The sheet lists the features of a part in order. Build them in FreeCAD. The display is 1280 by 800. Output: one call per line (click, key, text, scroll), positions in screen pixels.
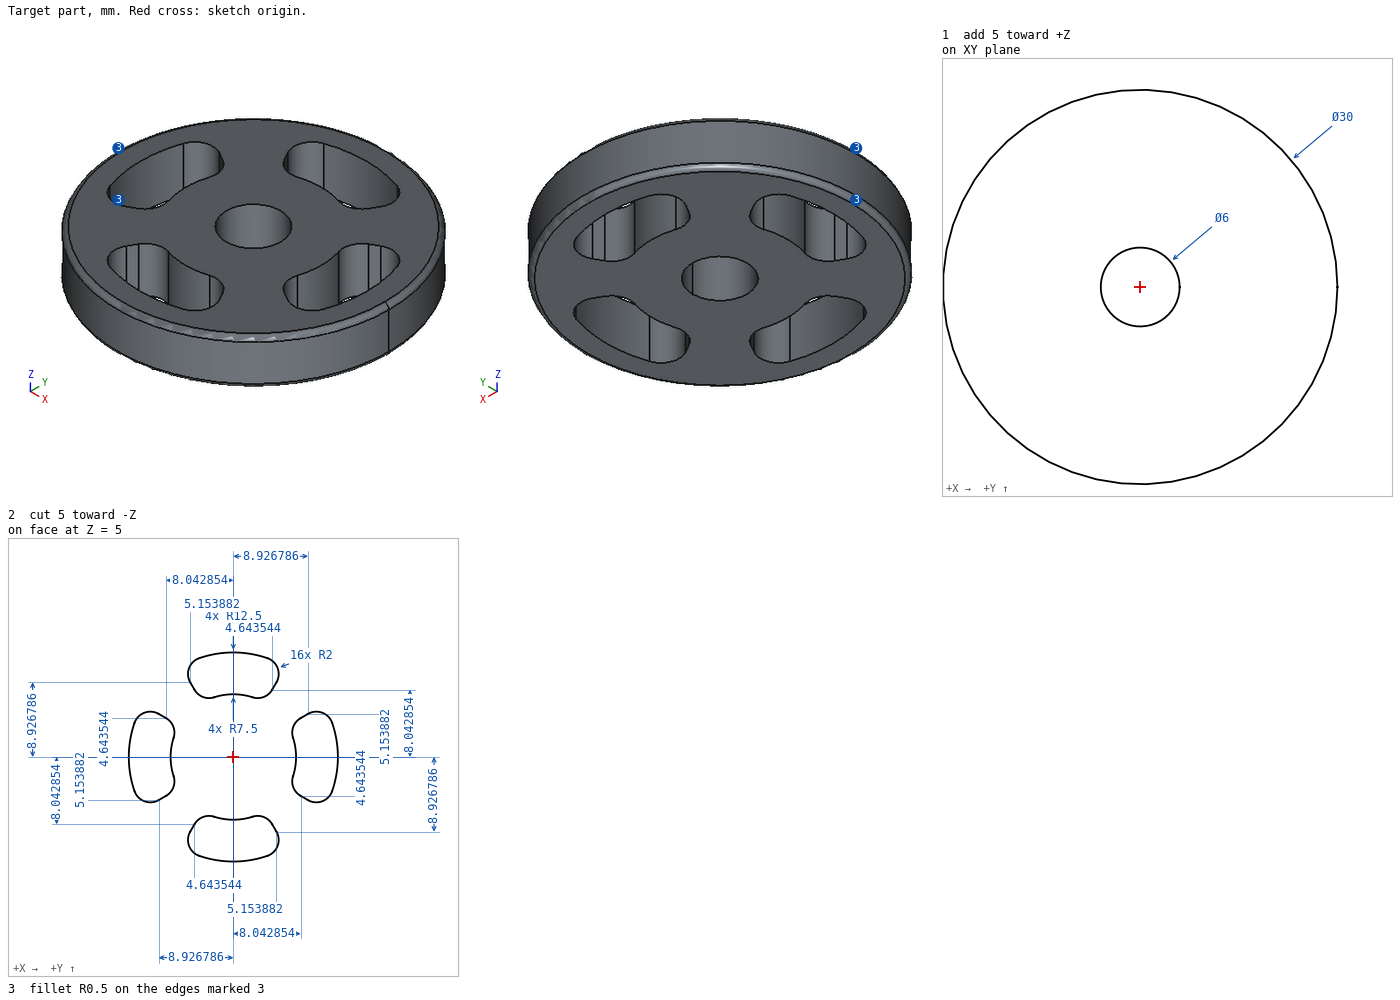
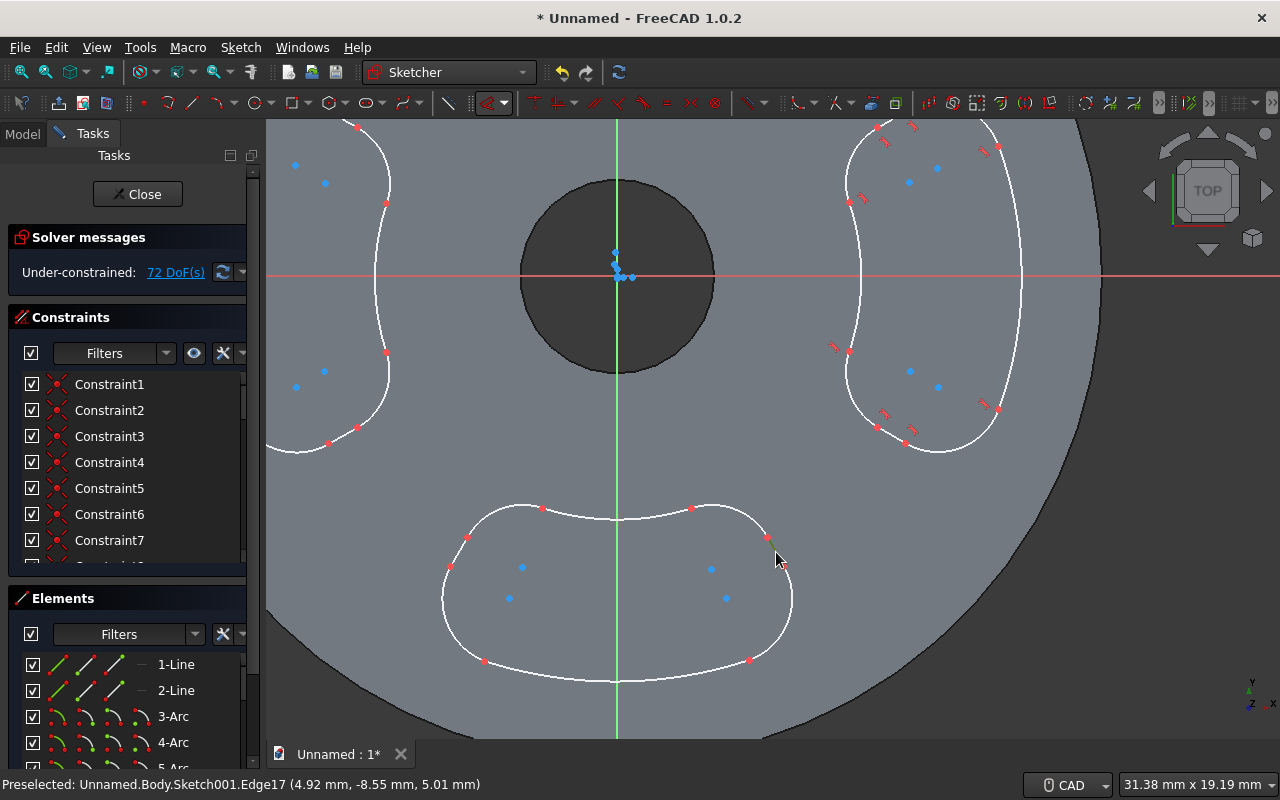
click(750, 518)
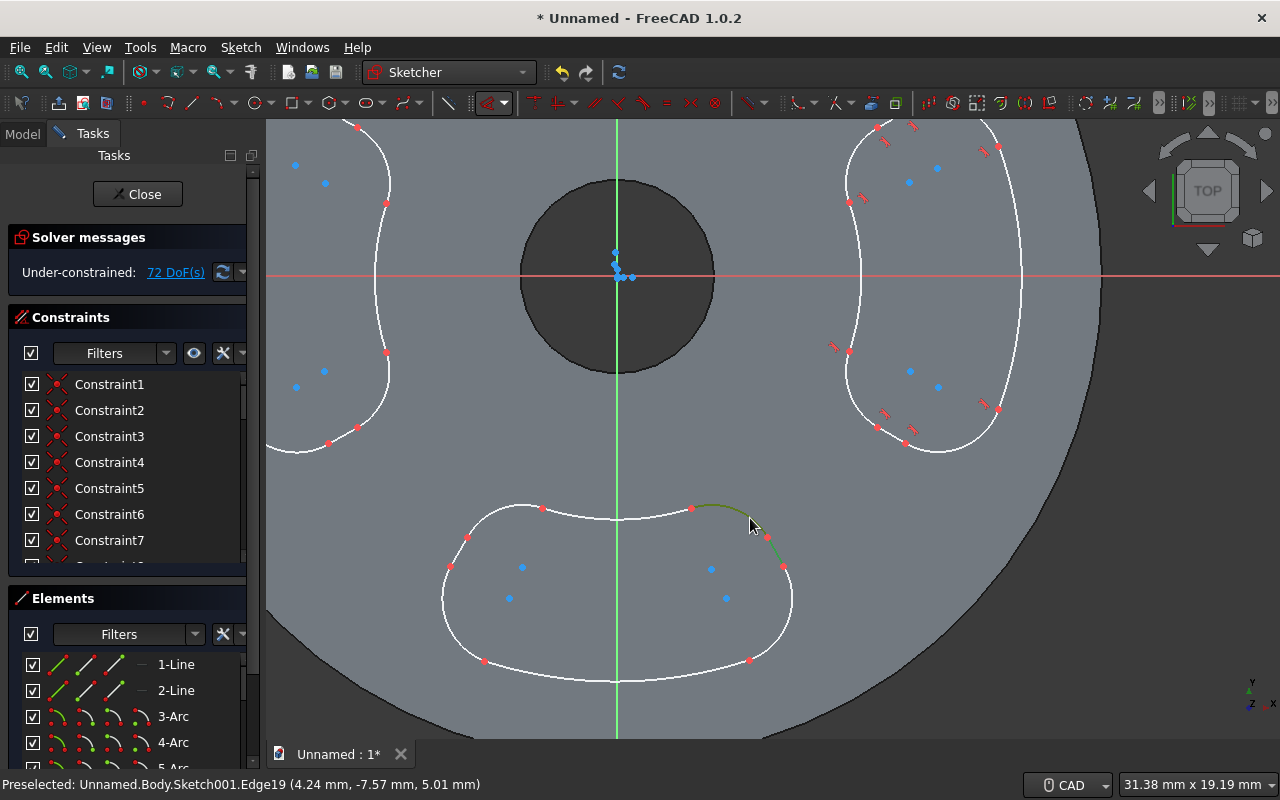
click(644, 104)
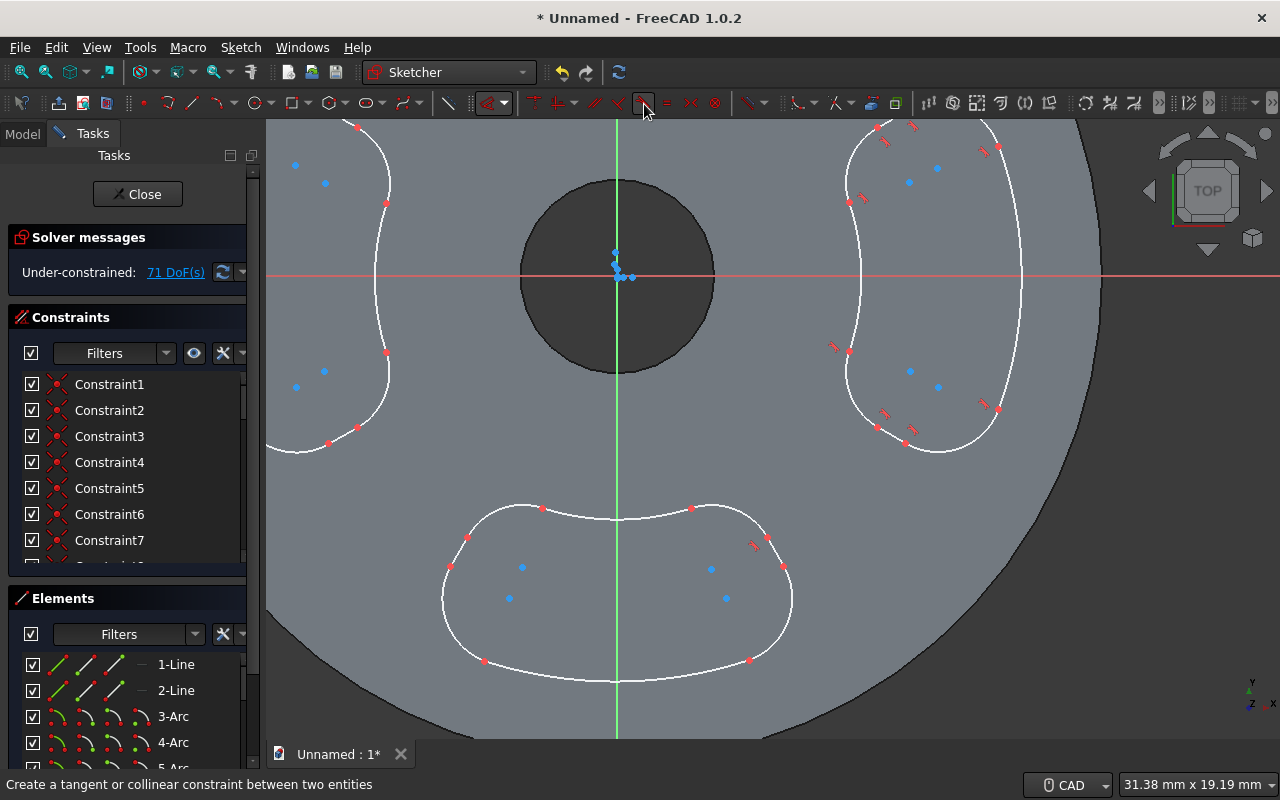
scroll(779, 558, up, 2)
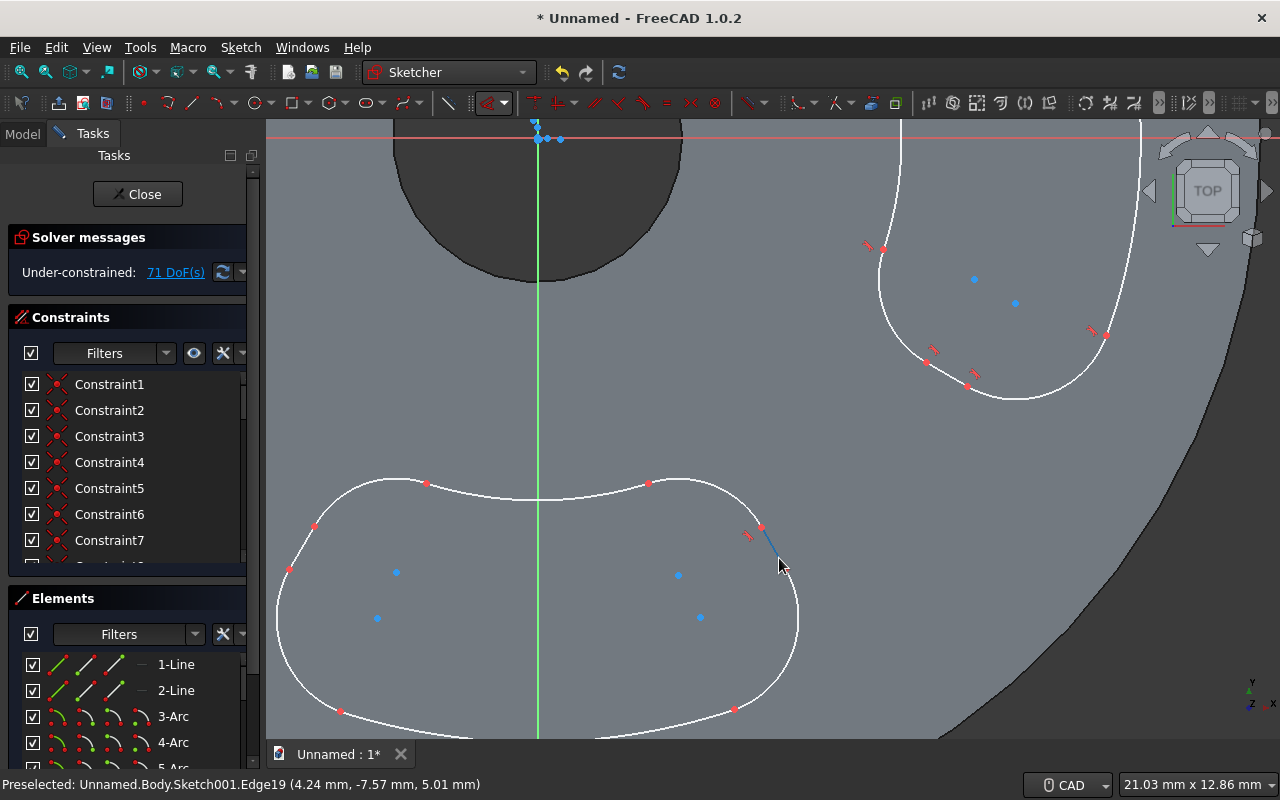
click(779, 557)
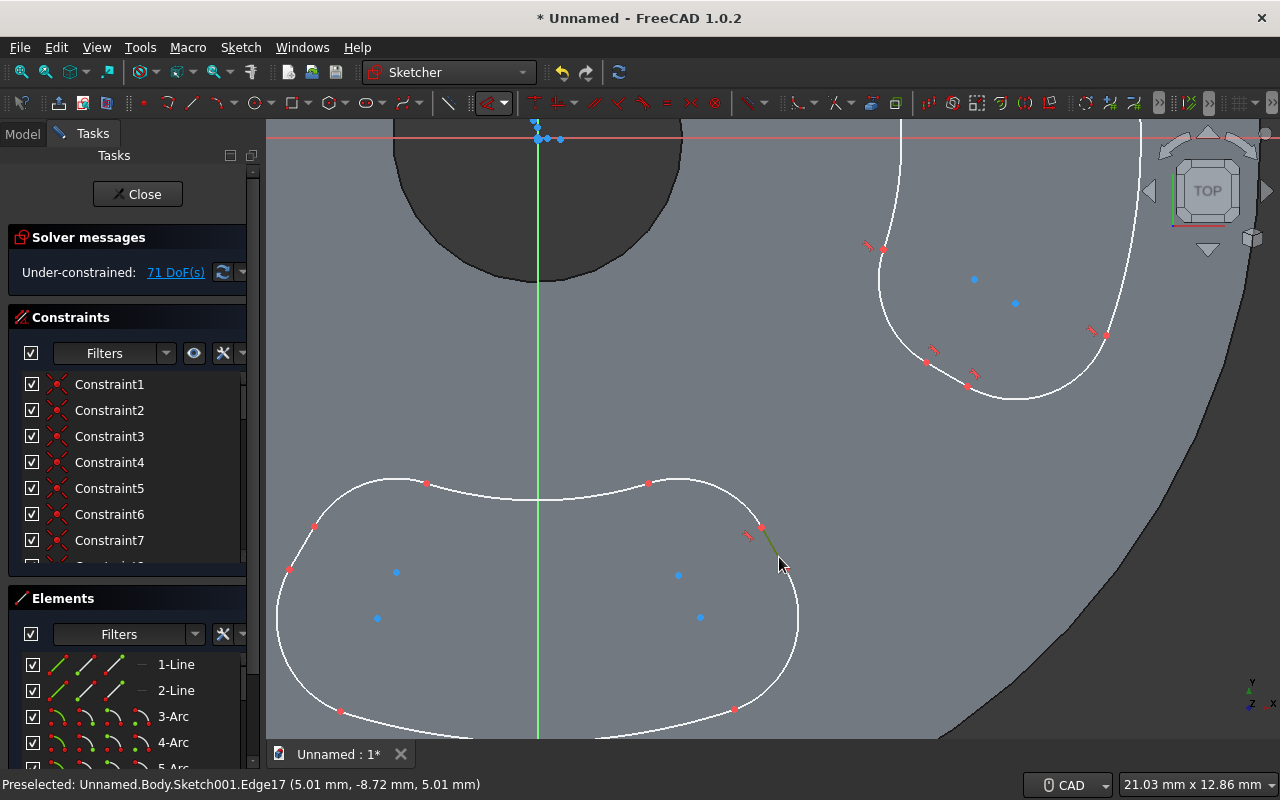
click(775, 681)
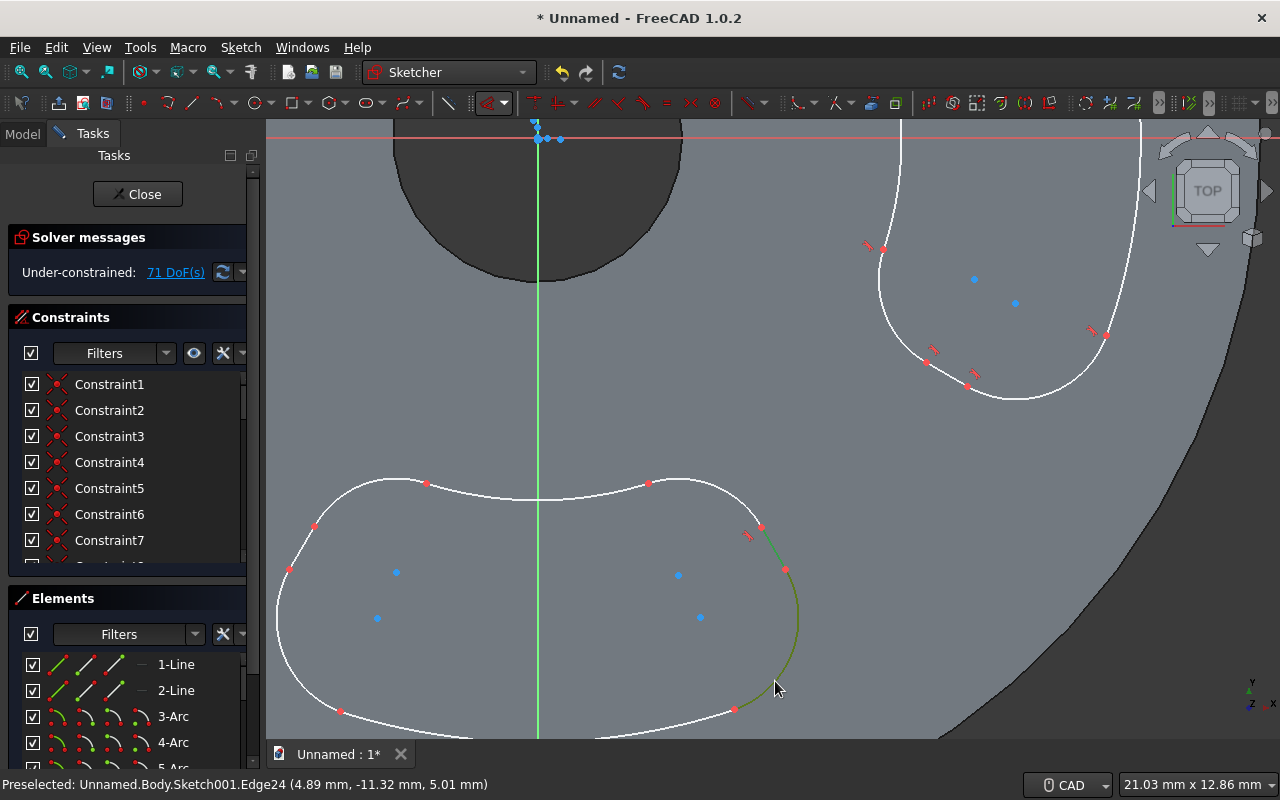
click(644, 104)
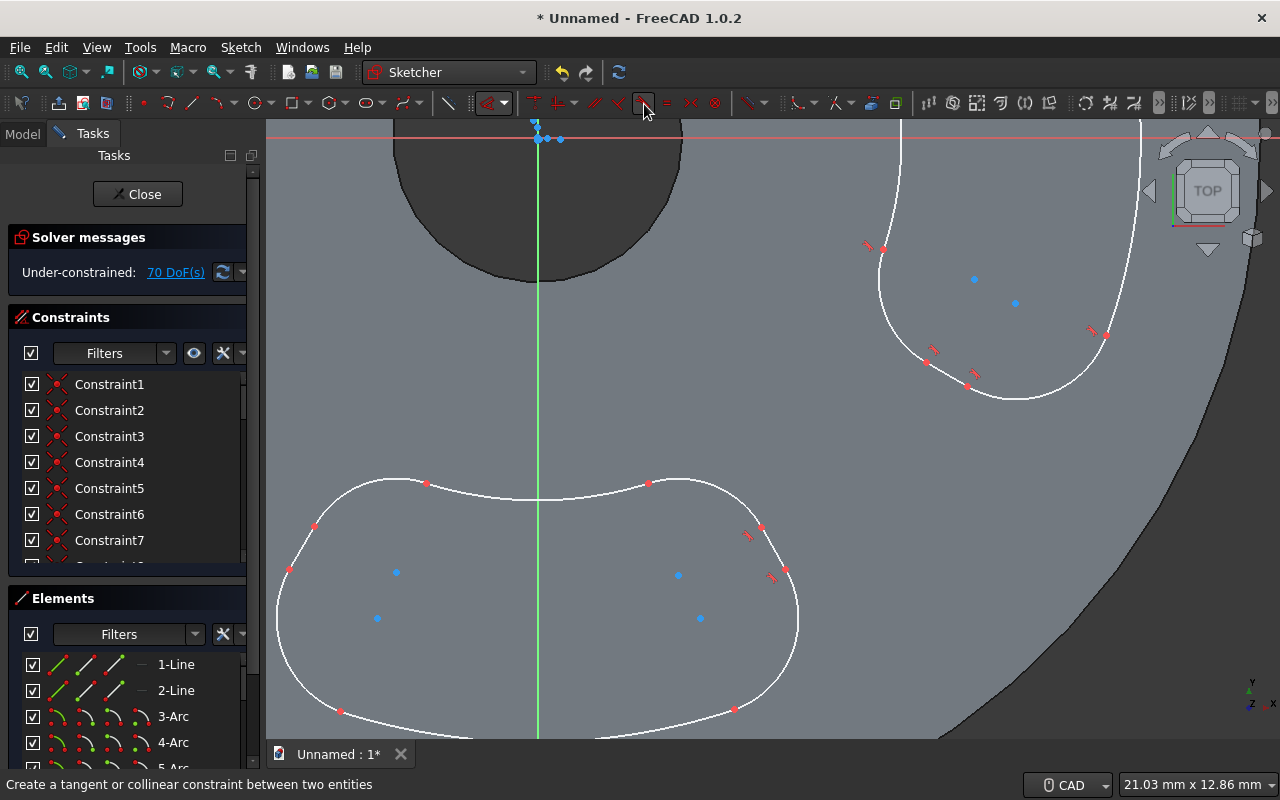
click(307, 540)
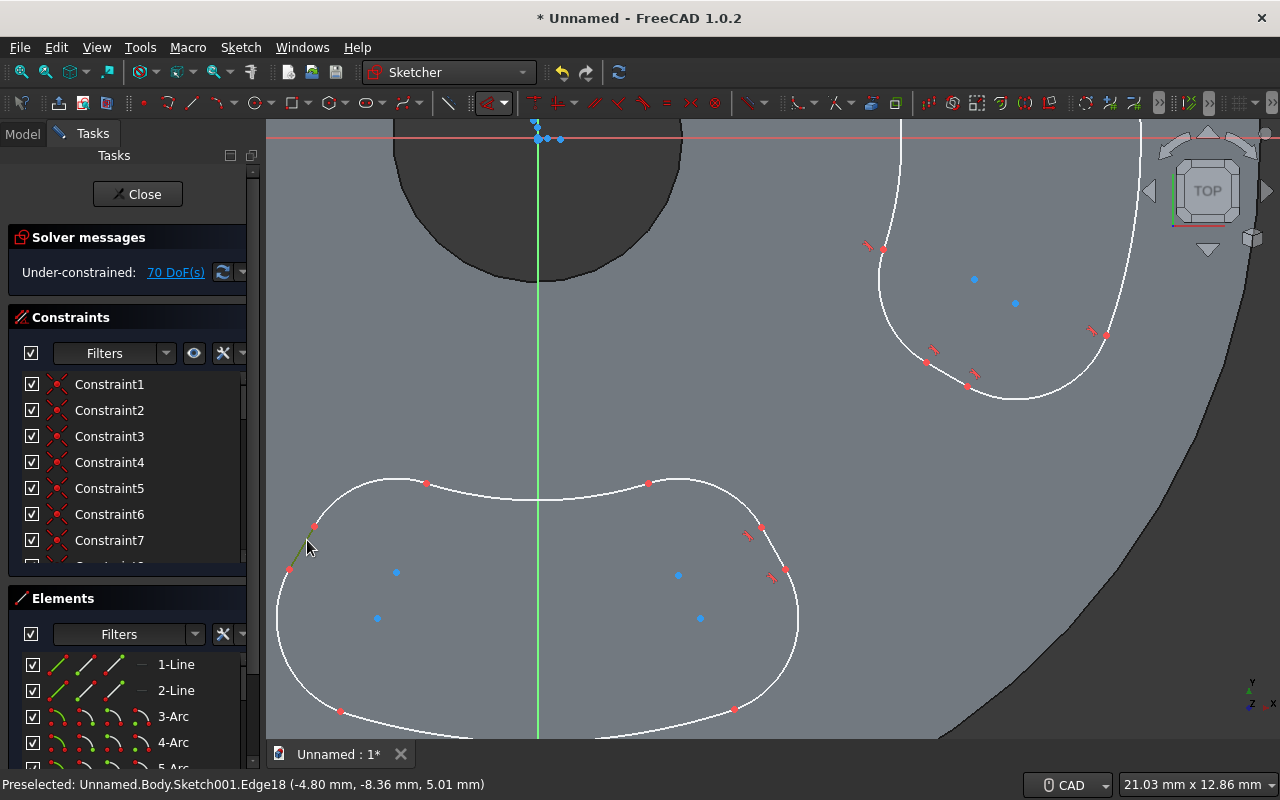
click(388, 479)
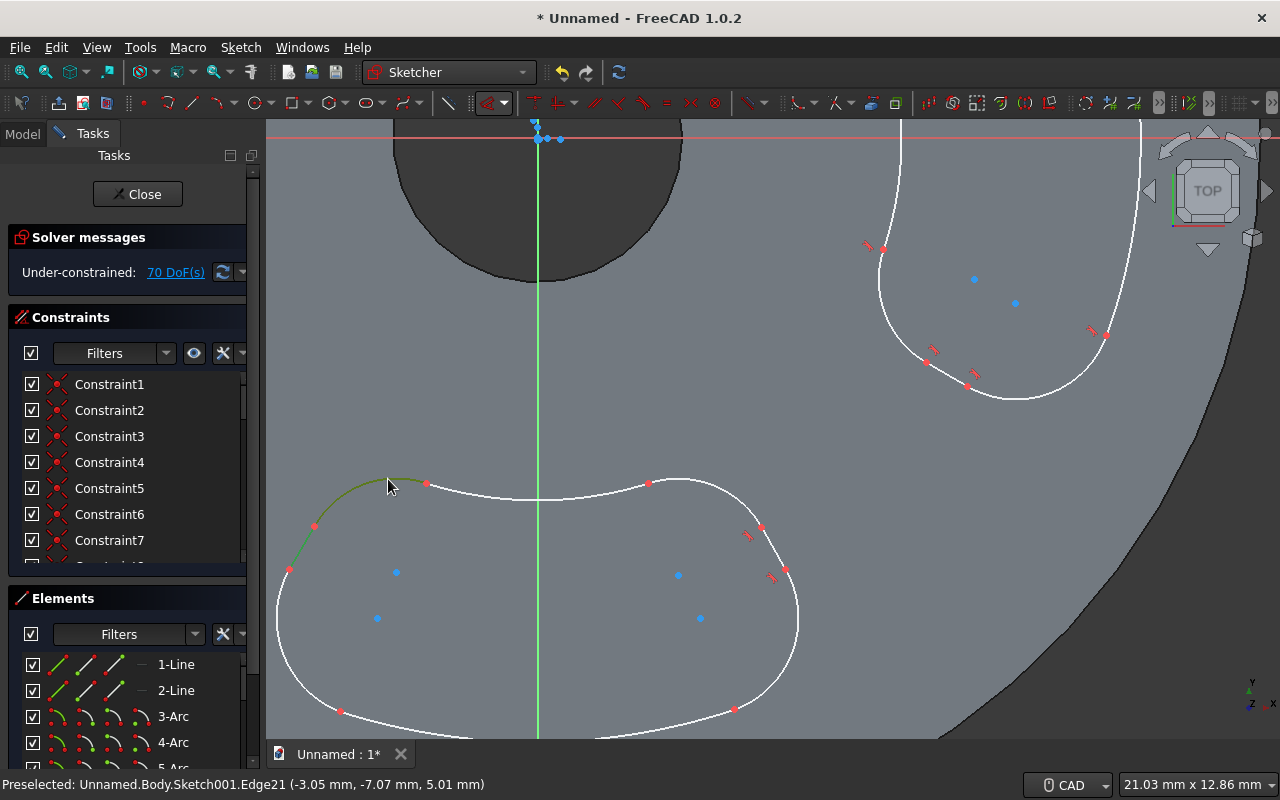
click(644, 104)